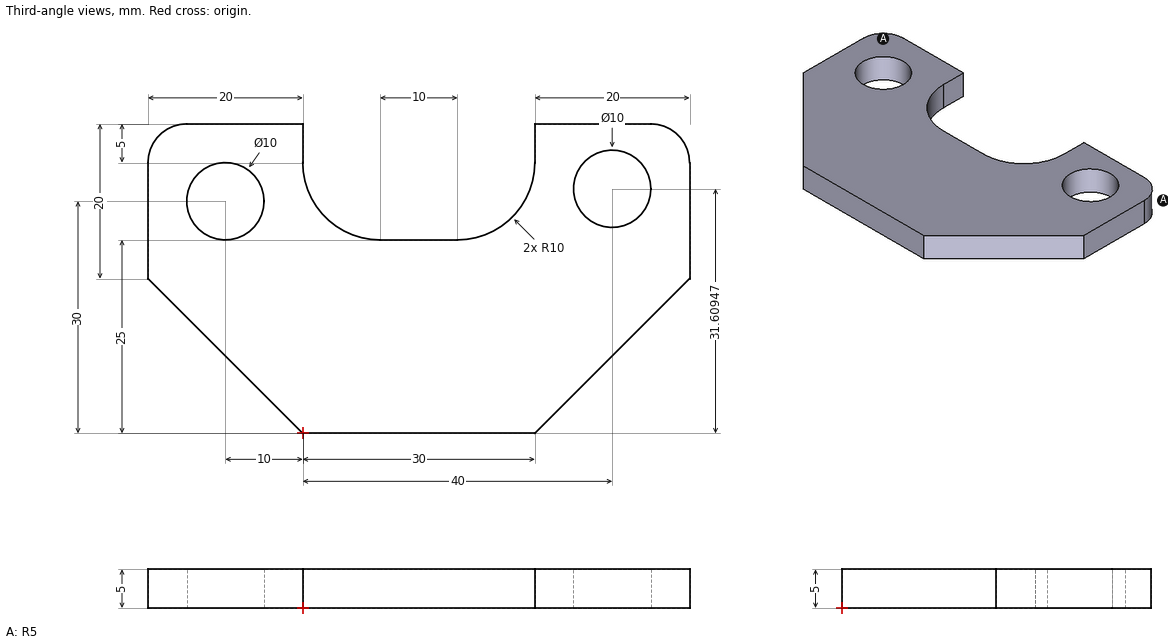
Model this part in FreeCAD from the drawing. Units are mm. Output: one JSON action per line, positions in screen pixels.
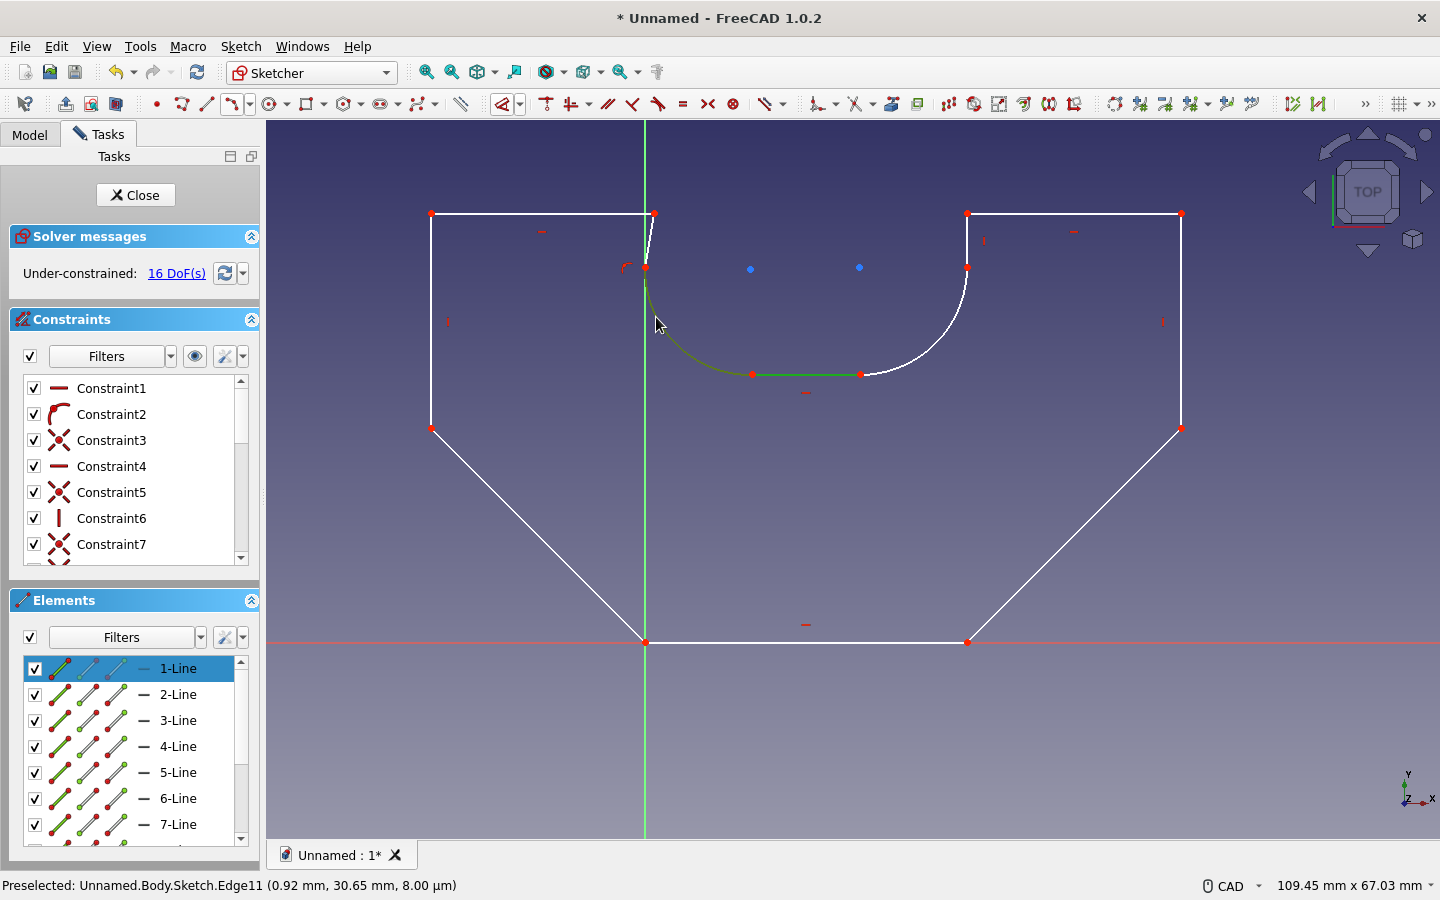
{"action": "left_click", "coordinate": [658, 104]}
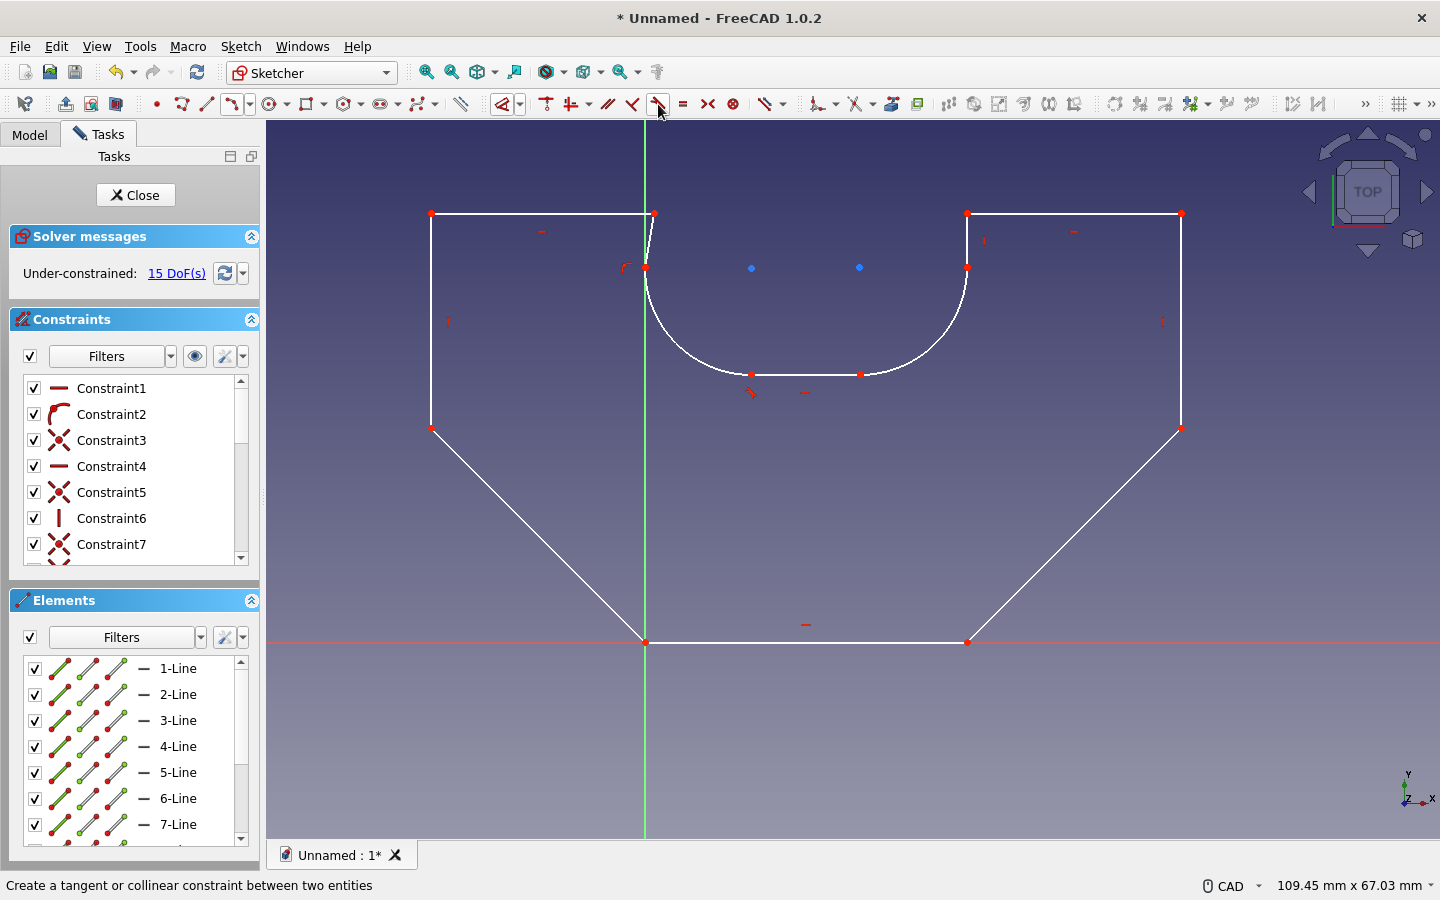
{"action": "left_click", "coordinate": [828, 375]}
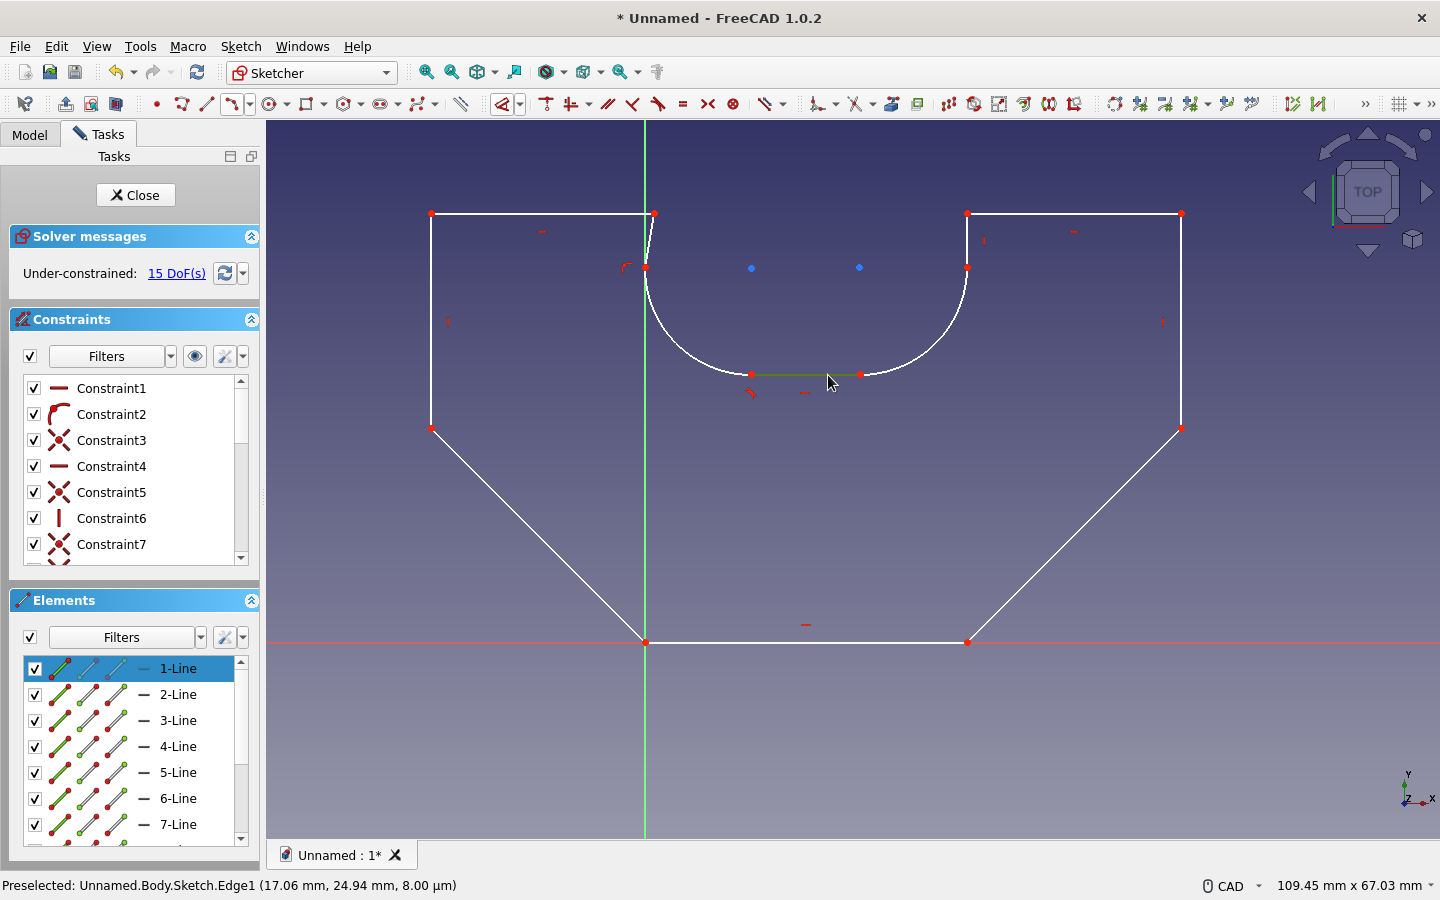
{"action": "left_click", "coordinate": [908, 363]}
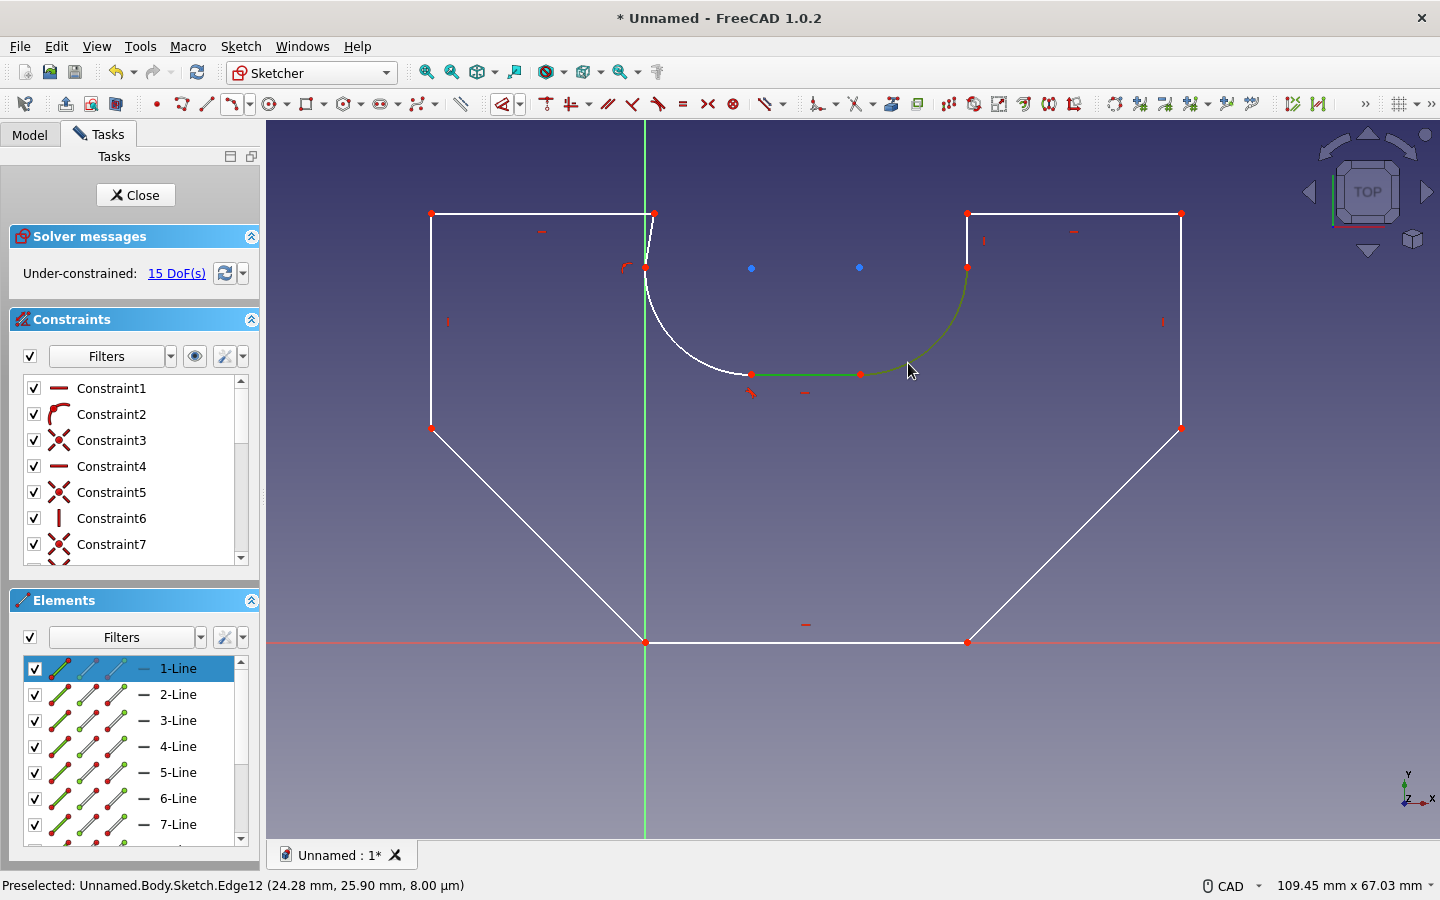
{"action": "left_click", "coordinate": [658, 104]}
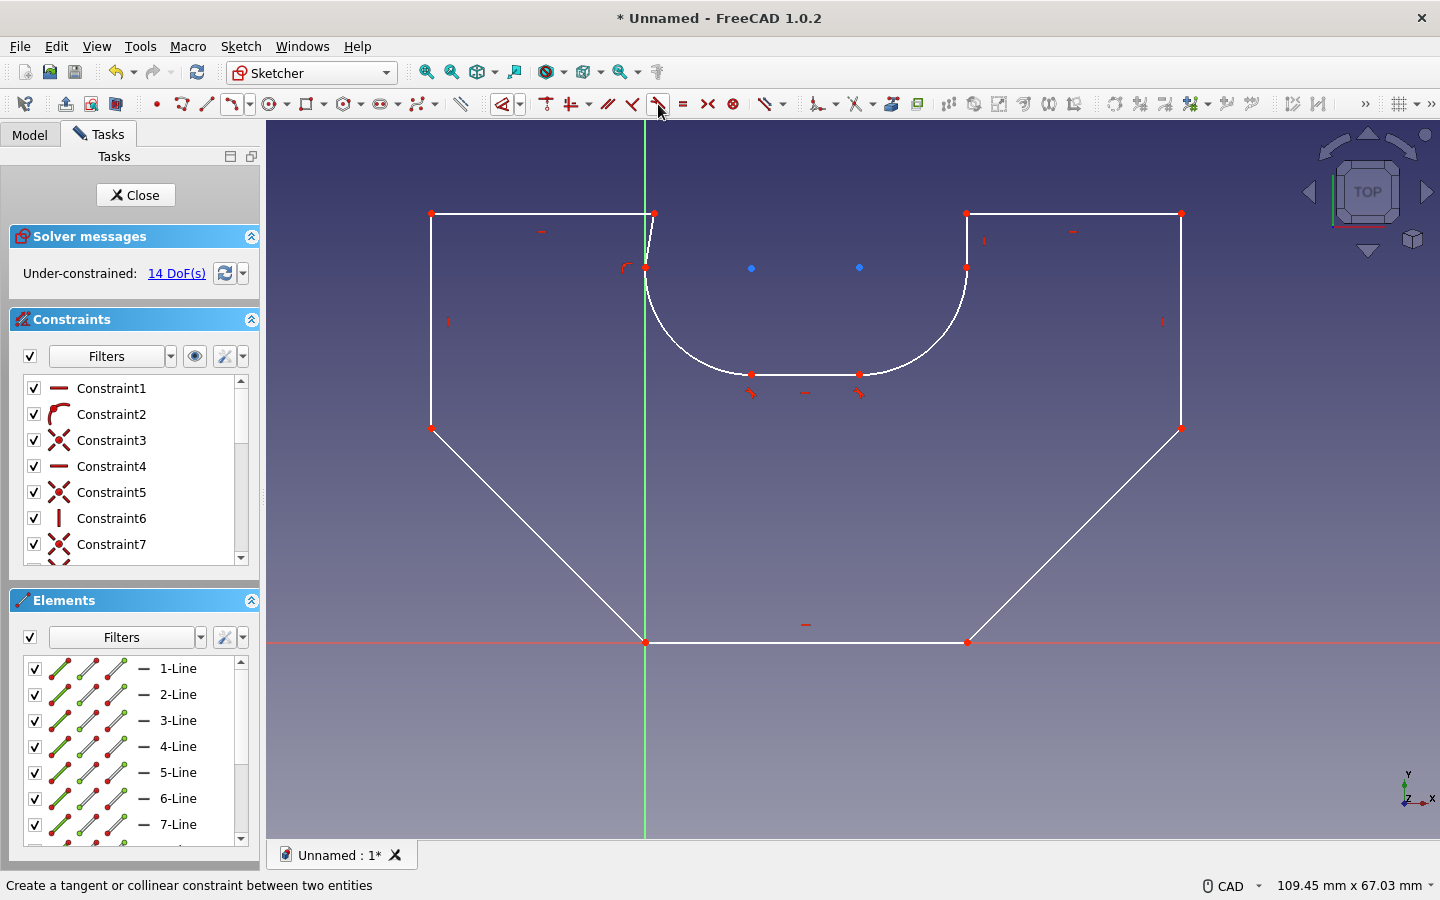
{"action": "left_click", "coordinate": [648, 252]}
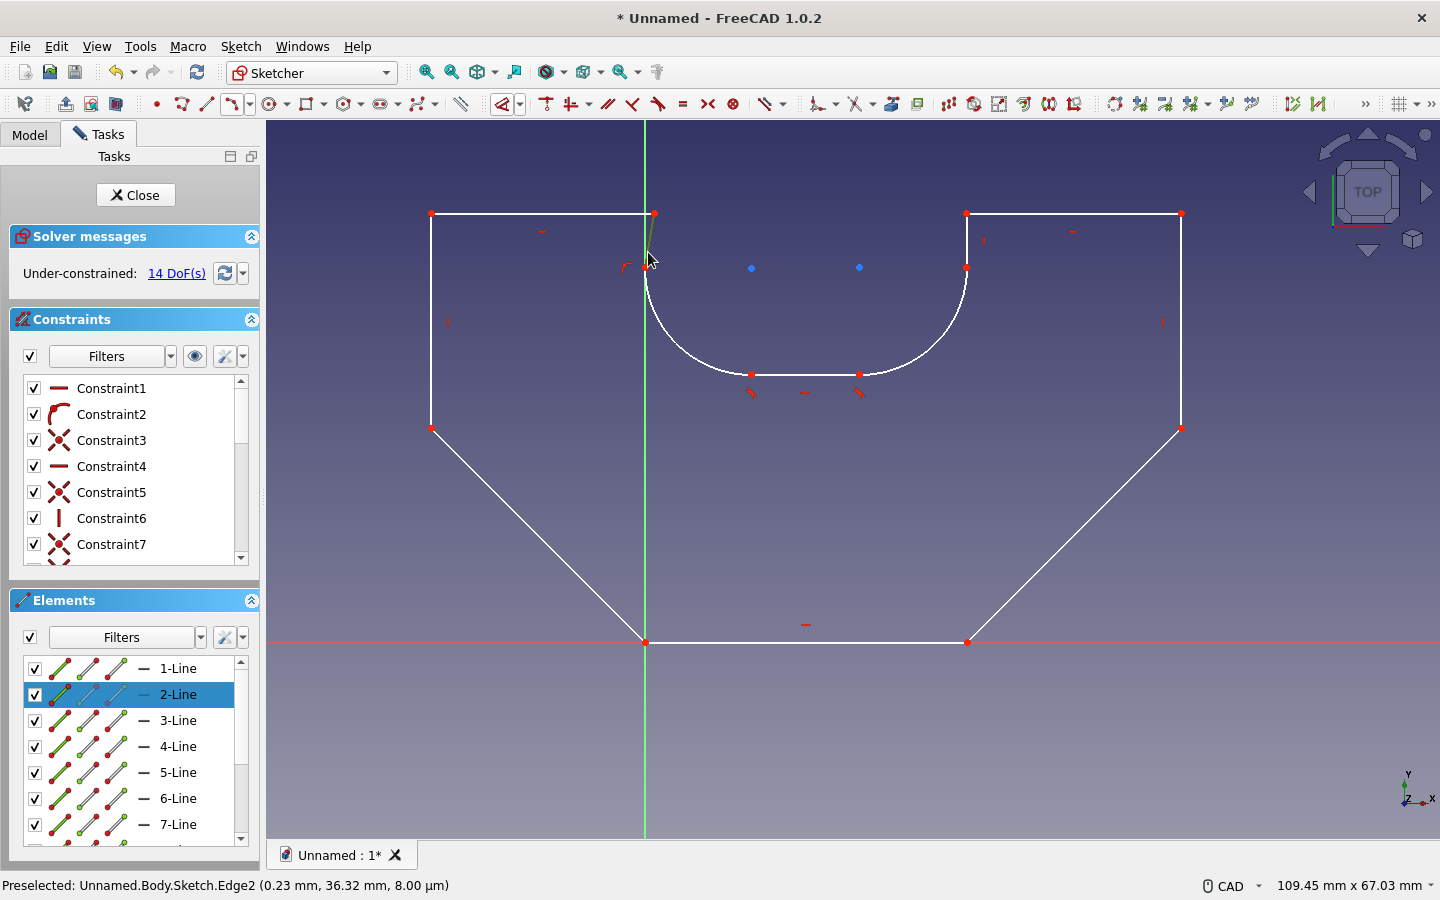
{"action": "left_click", "coordinate": [657, 317]}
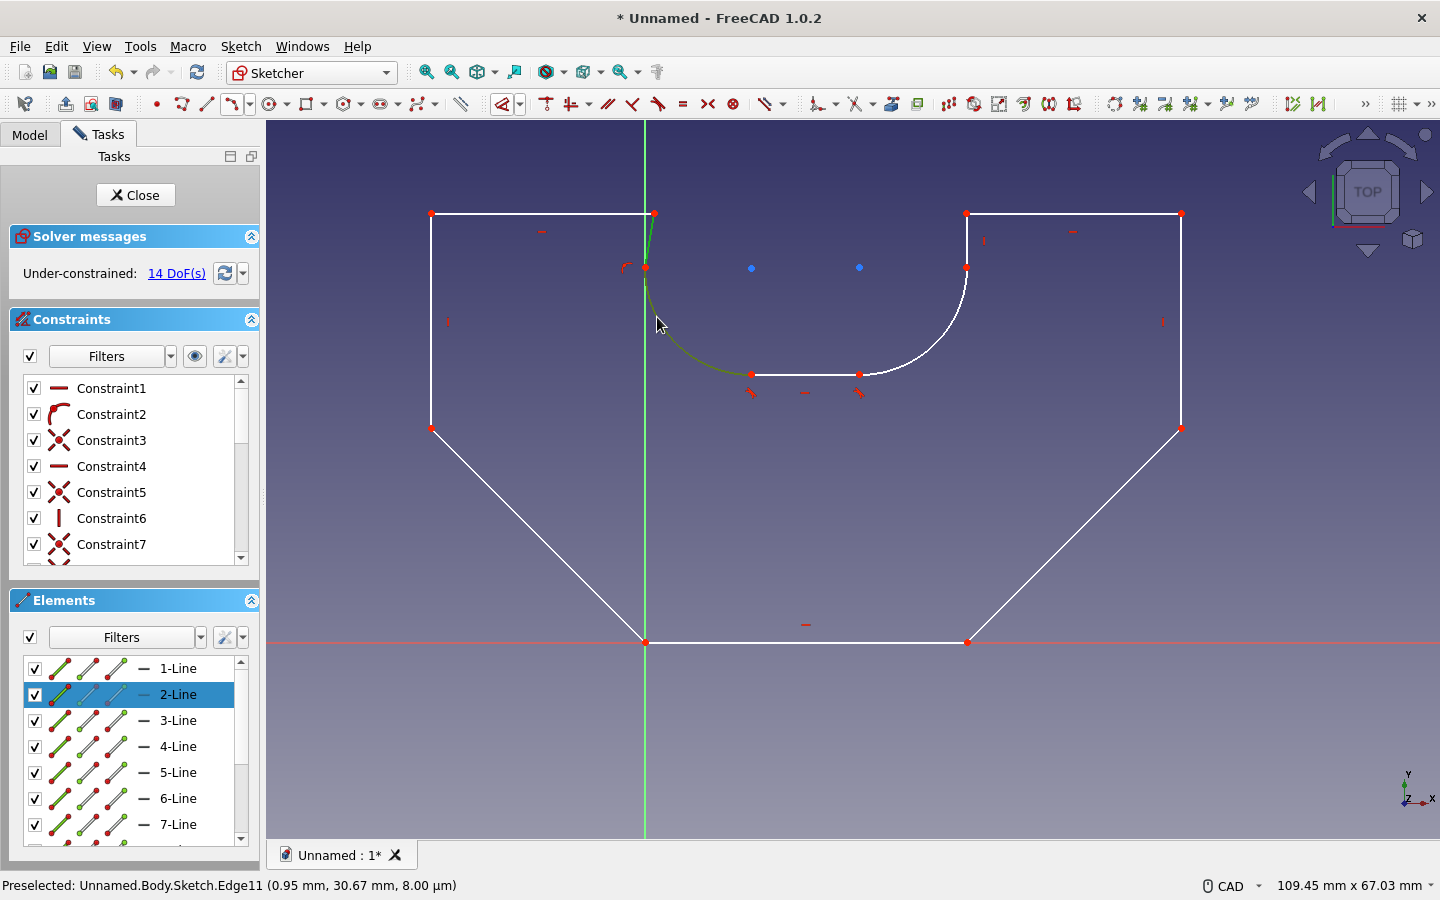
{"action": "left_click", "coordinate": [658, 104]}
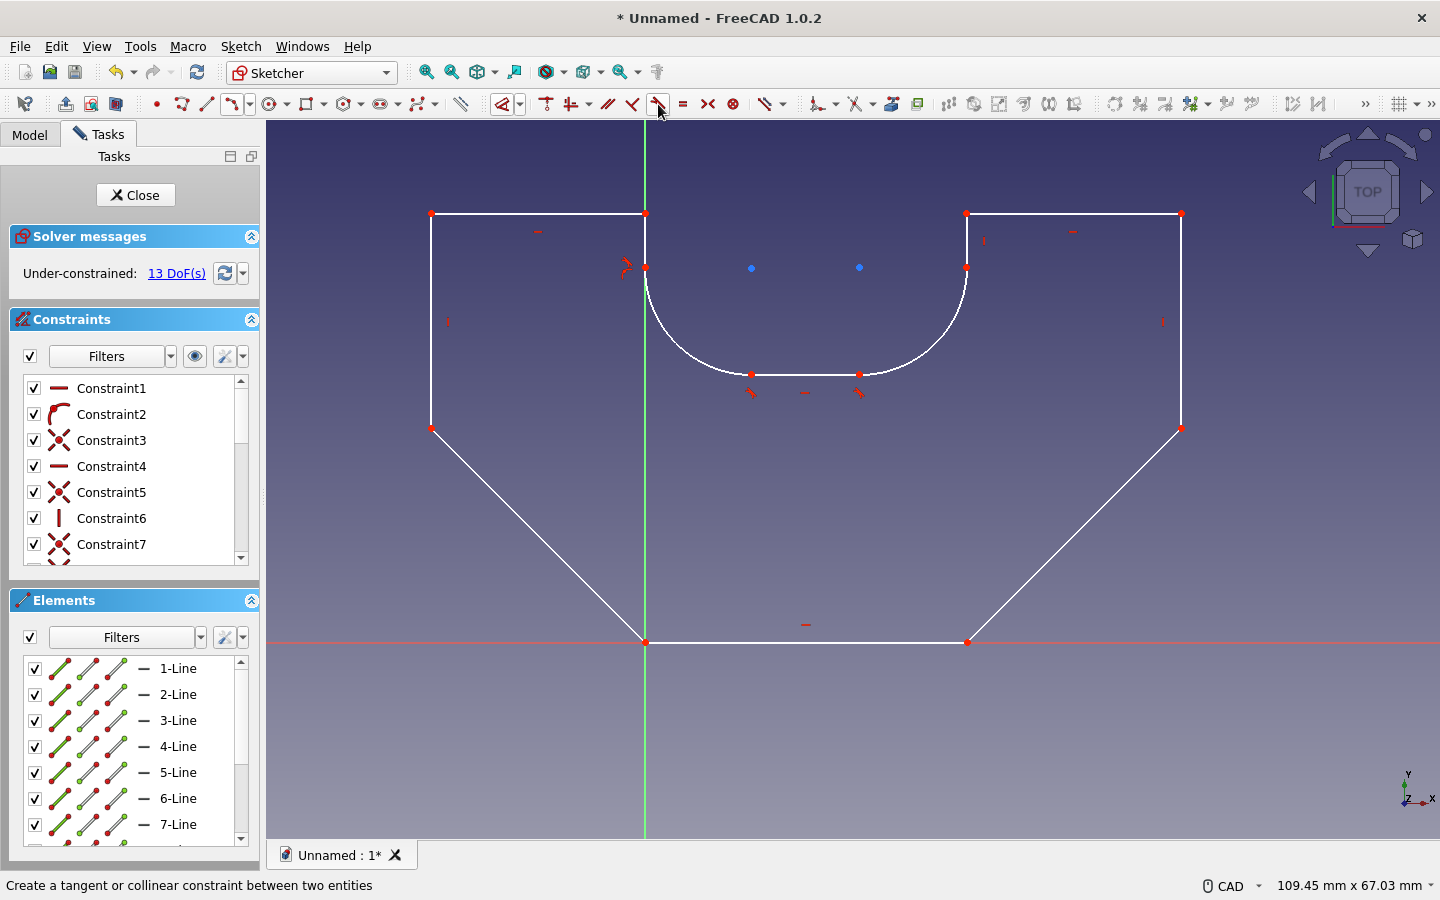
{"action": "left_click", "coordinate": [967, 230]}